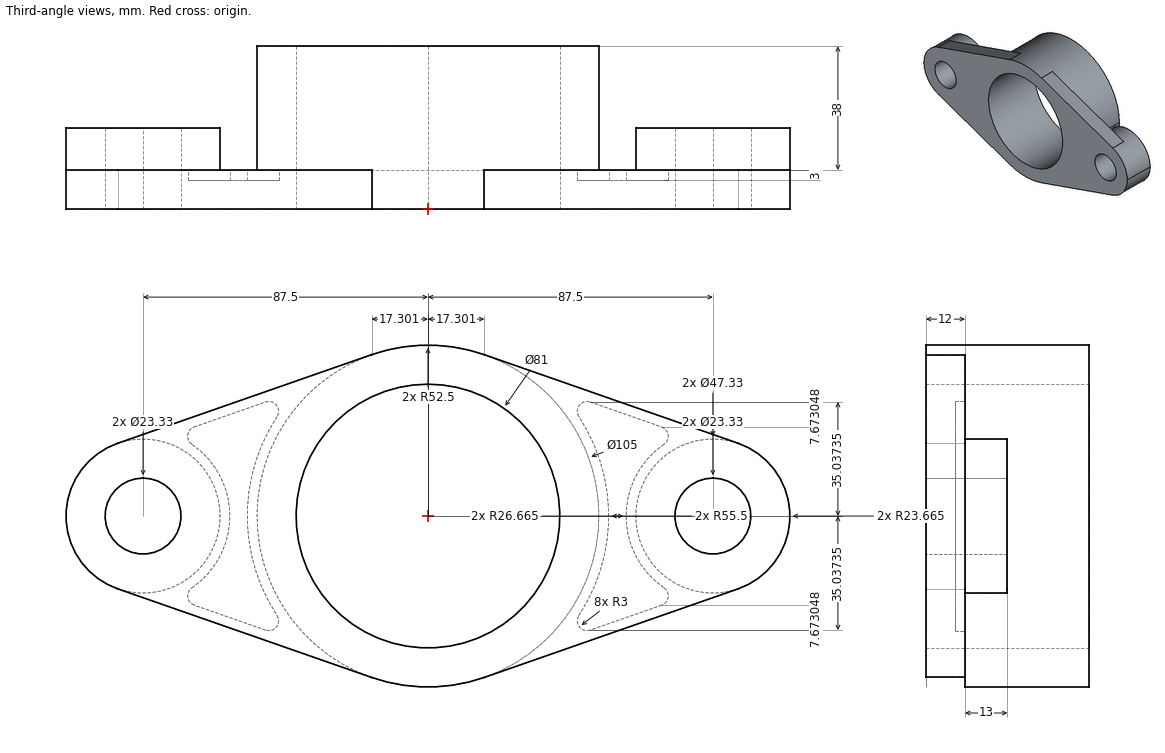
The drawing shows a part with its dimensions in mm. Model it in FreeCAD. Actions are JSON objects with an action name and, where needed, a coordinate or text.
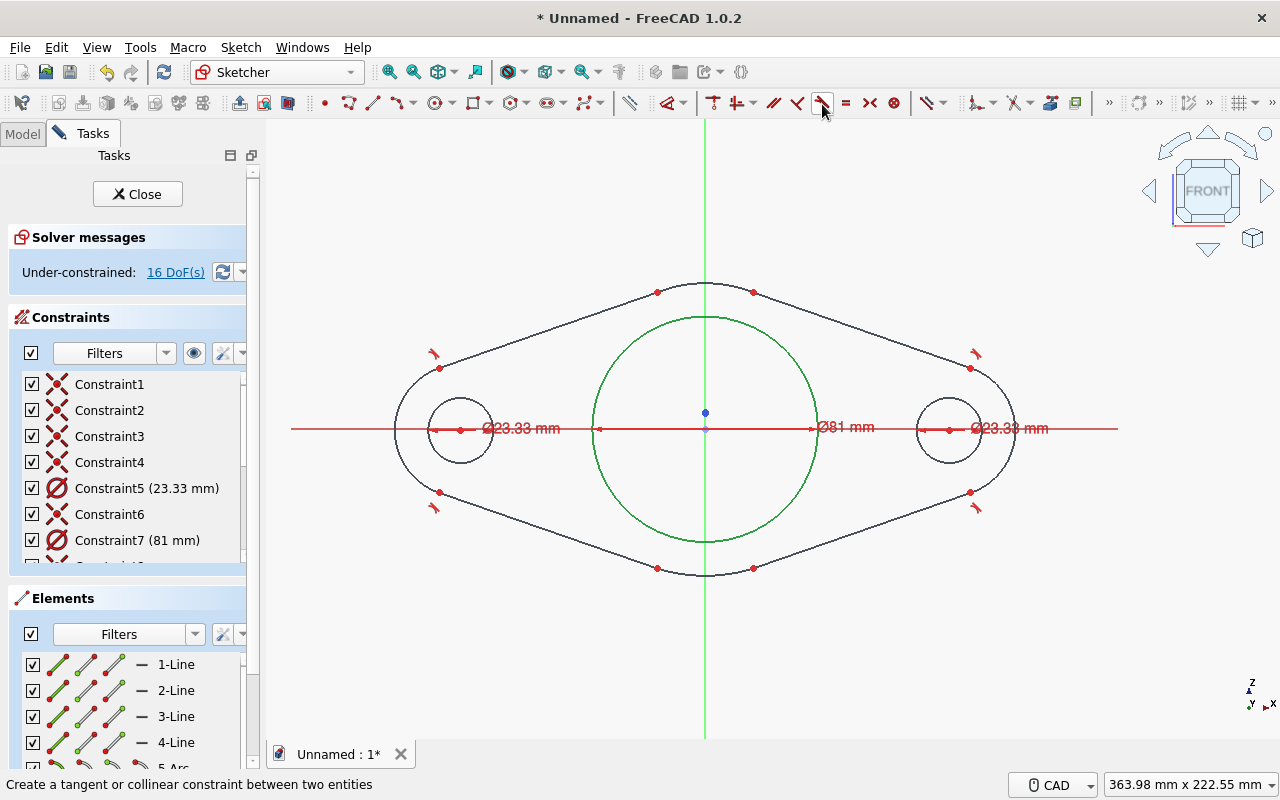
{"action": "left_click", "coordinate": [785, 349]}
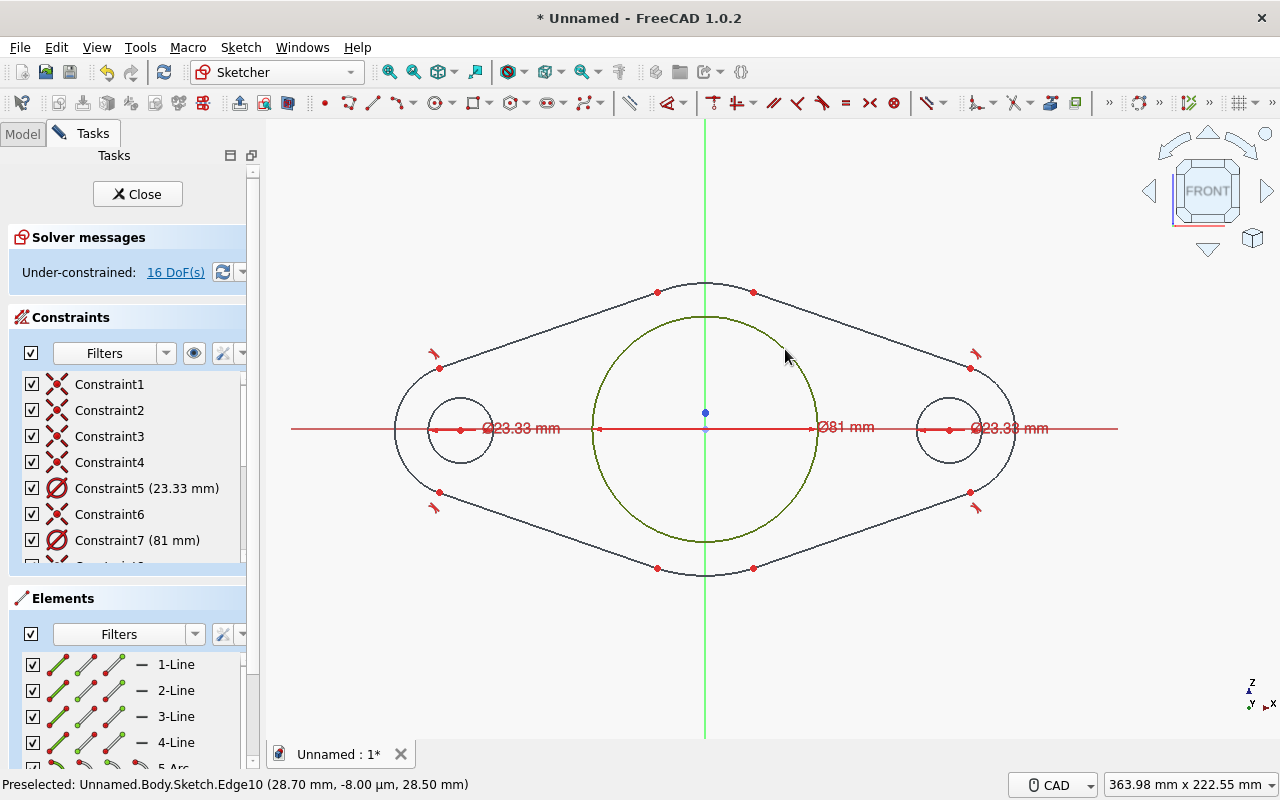
{"action": "left_click", "coordinate": [725, 285]}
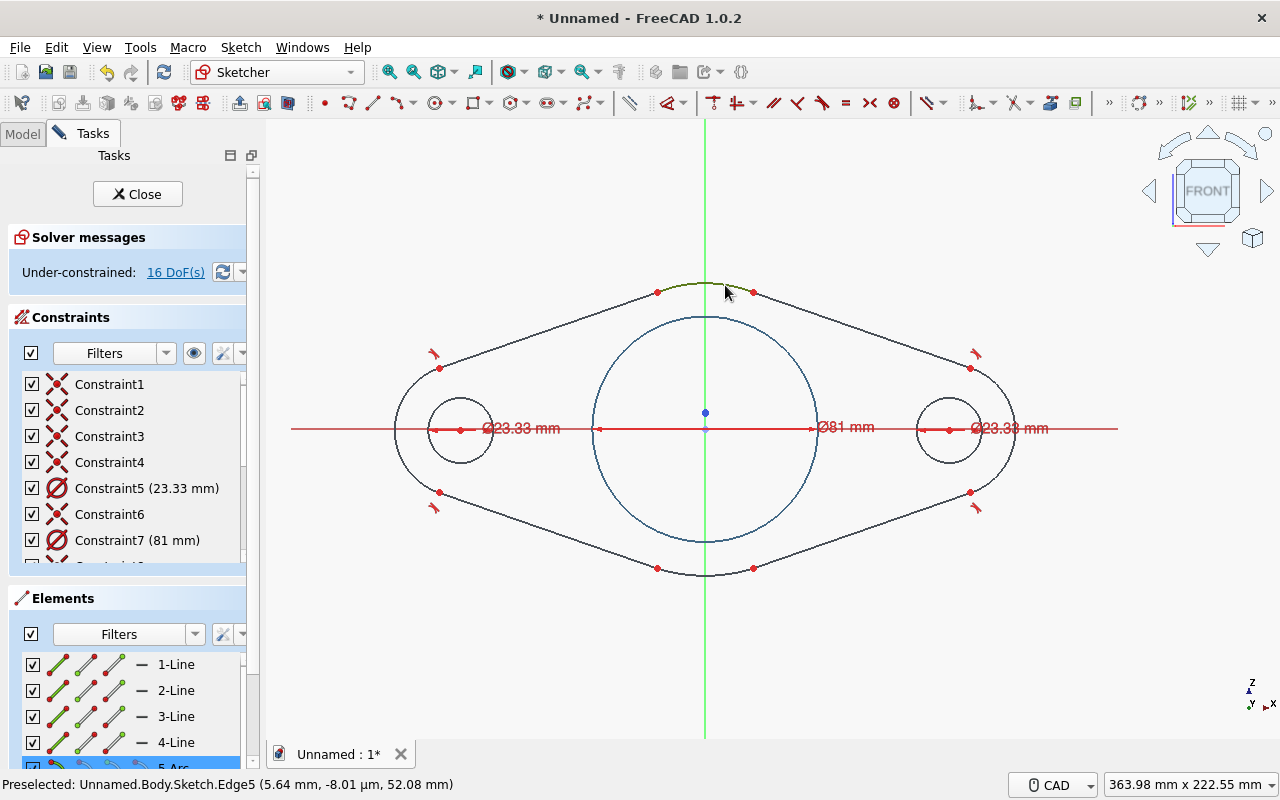
{"action": "left_click", "coordinate": [714, 104]}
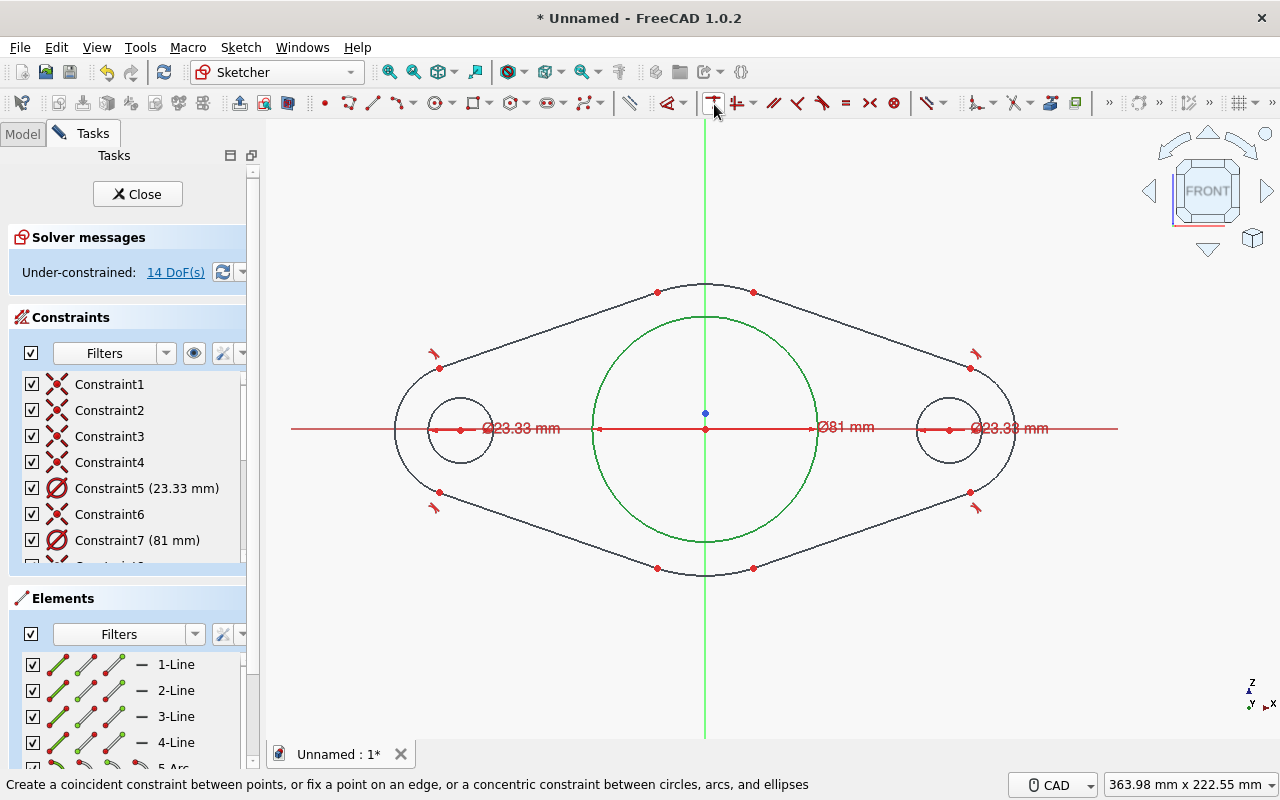
{"action": "left_click", "coordinate": [785, 349]}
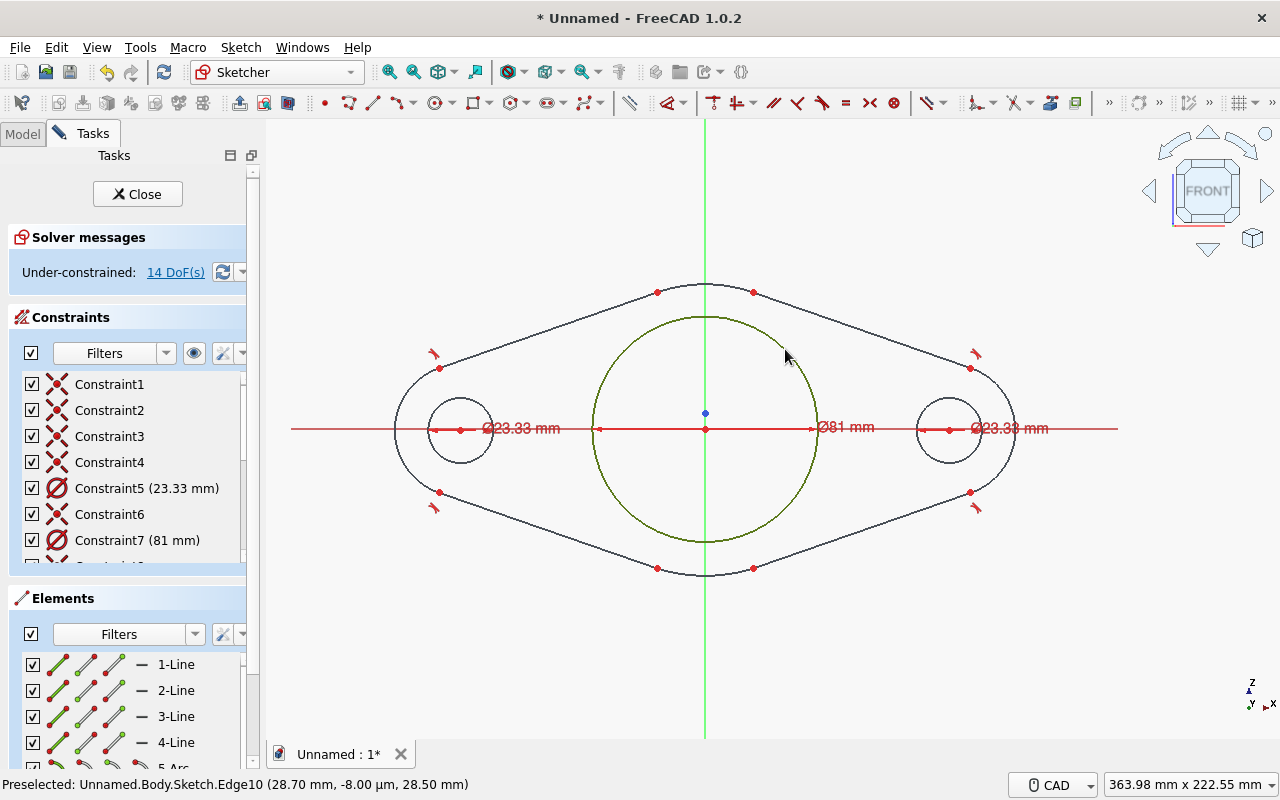
{"action": "left_click", "coordinate": [686, 575]}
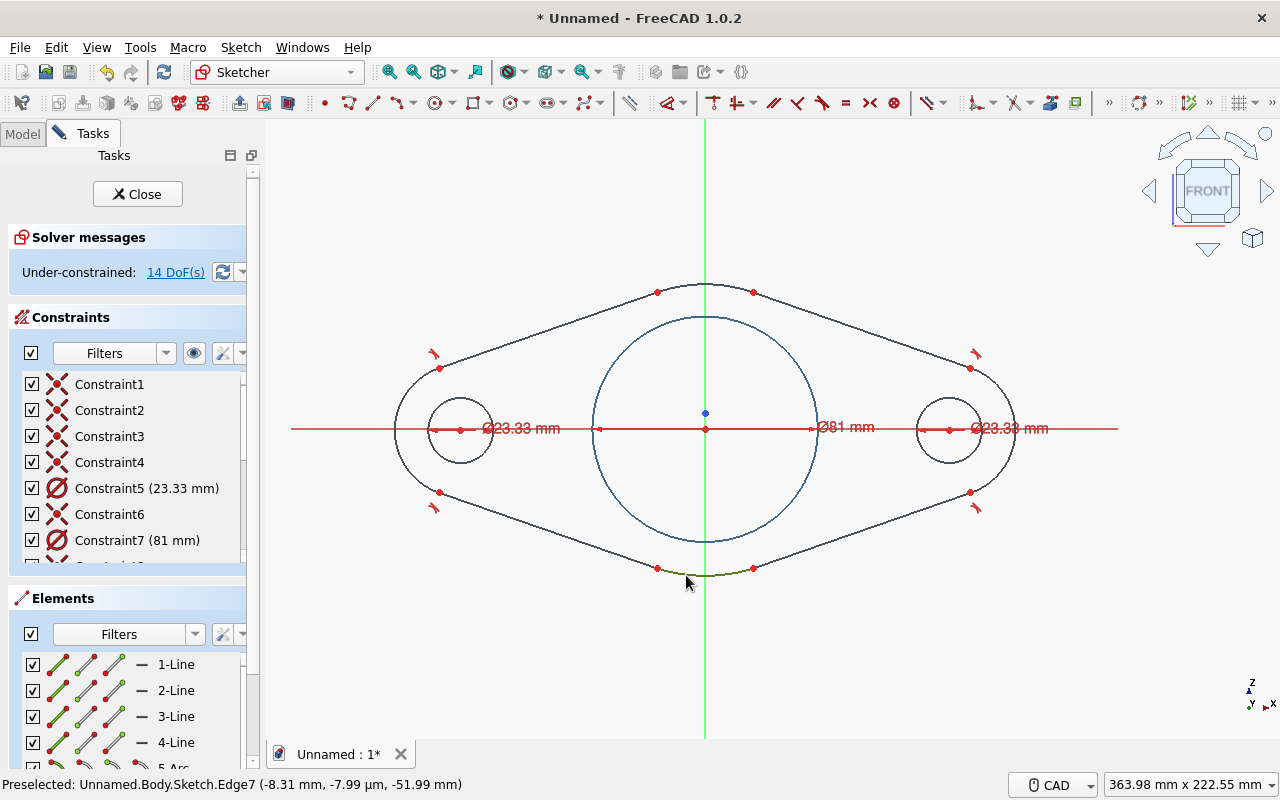
{"action": "left_click", "coordinate": [714, 104]}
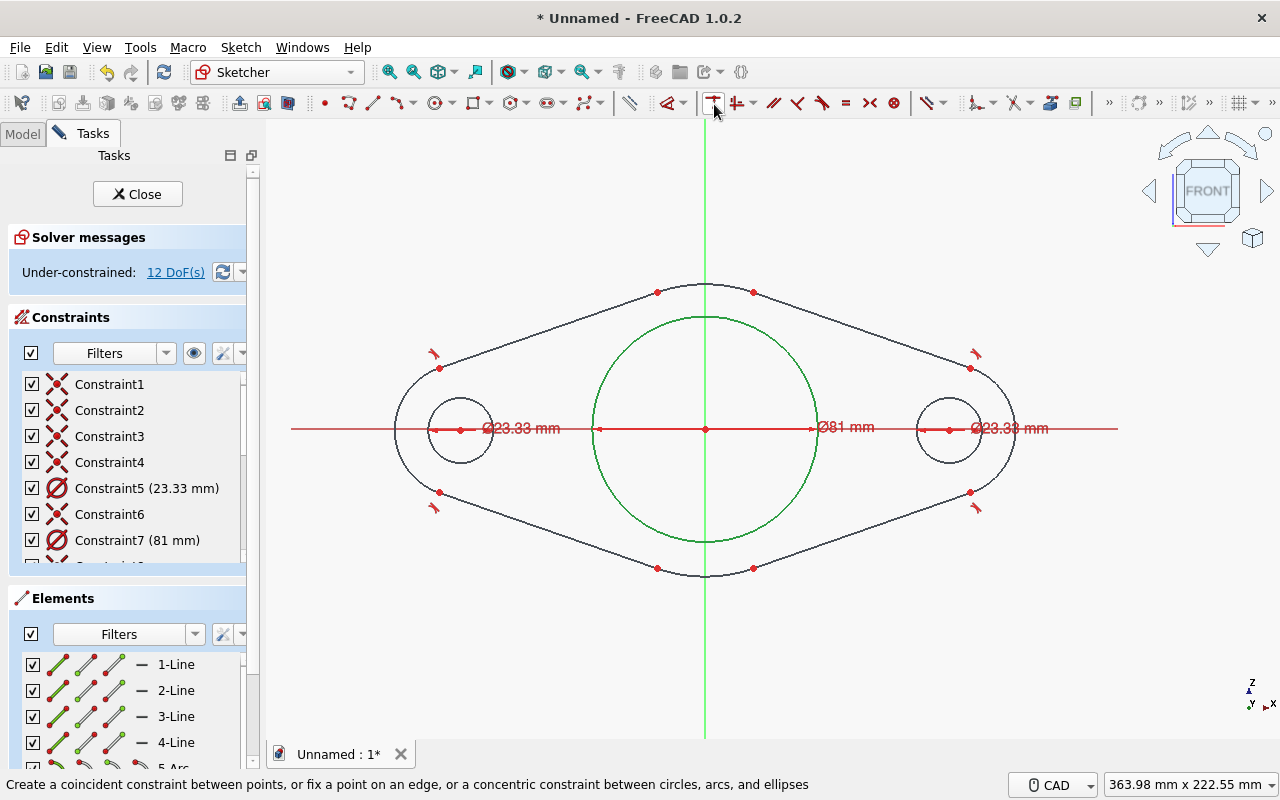
{"action": "left_click", "coordinate": [725, 286]}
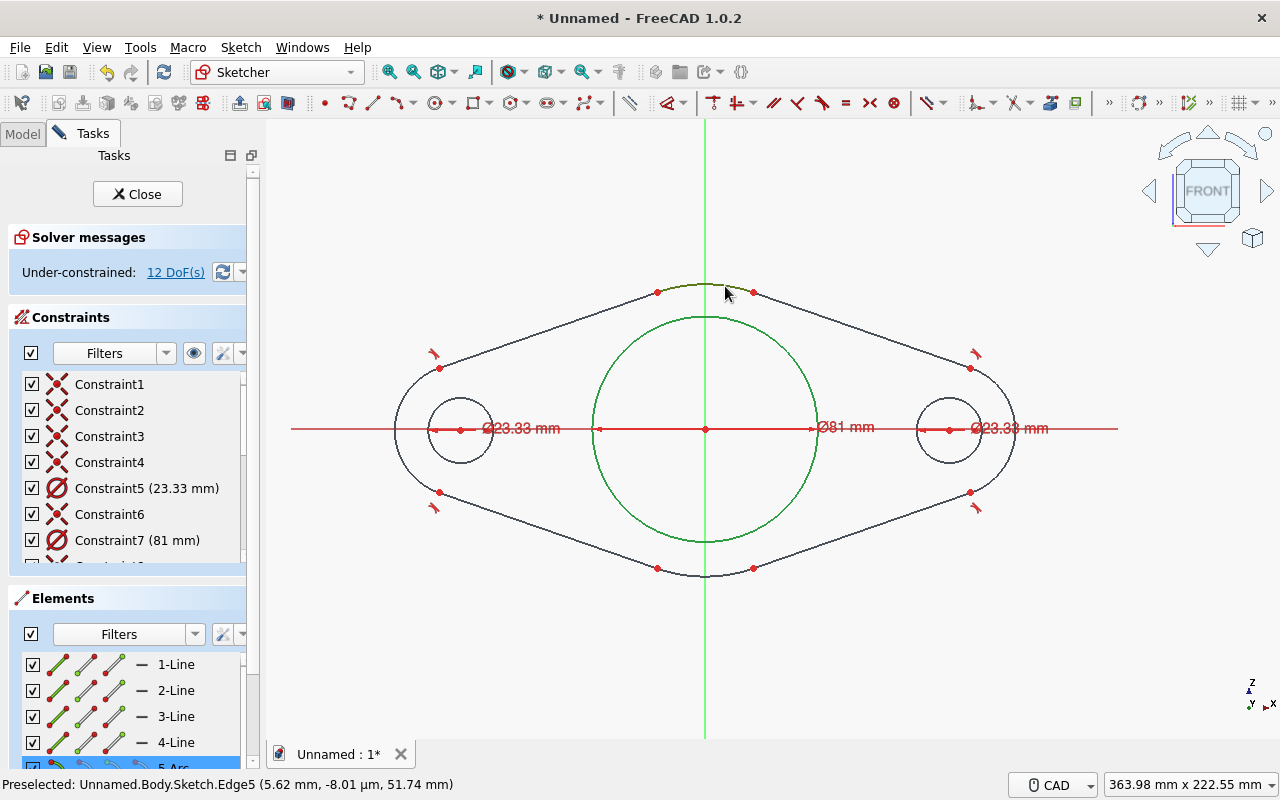
{"action": "left_click", "coordinate": [686, 575]}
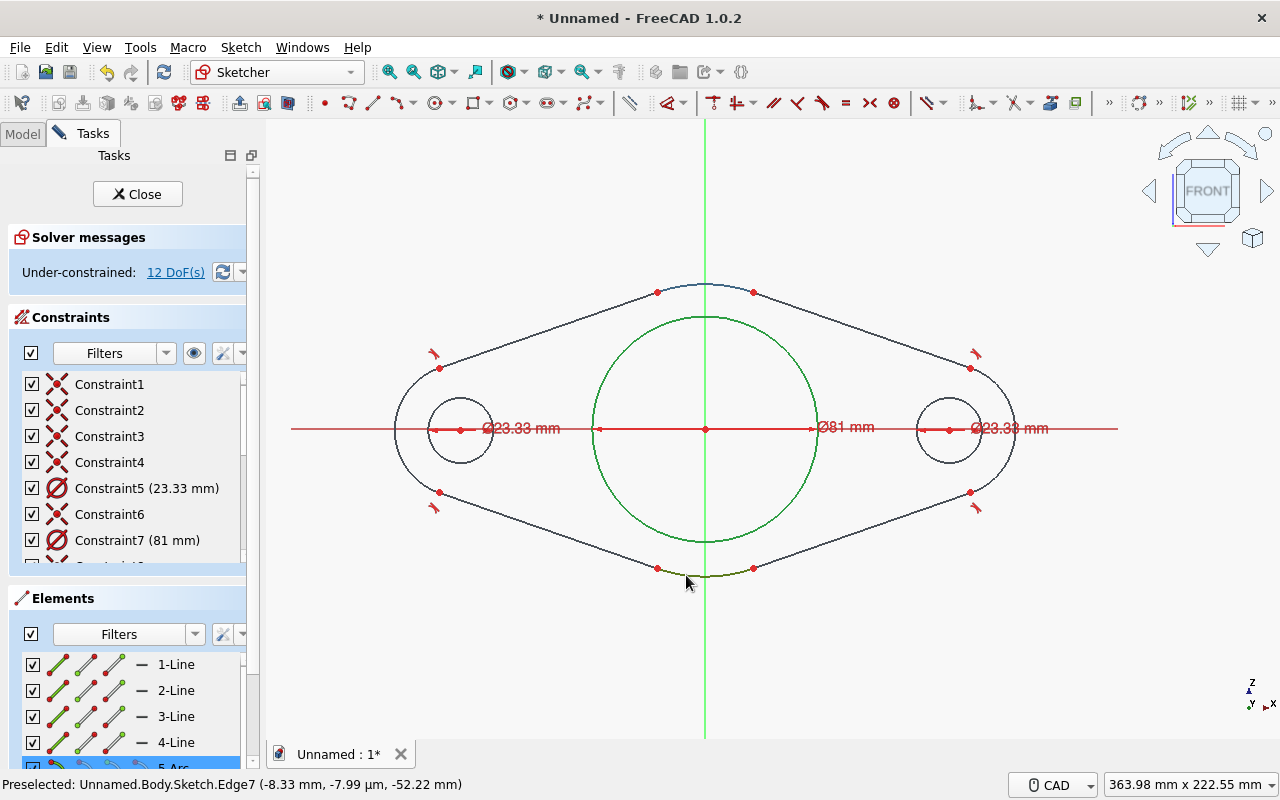
{"action": "left_click", "coordinate": [846, 104]}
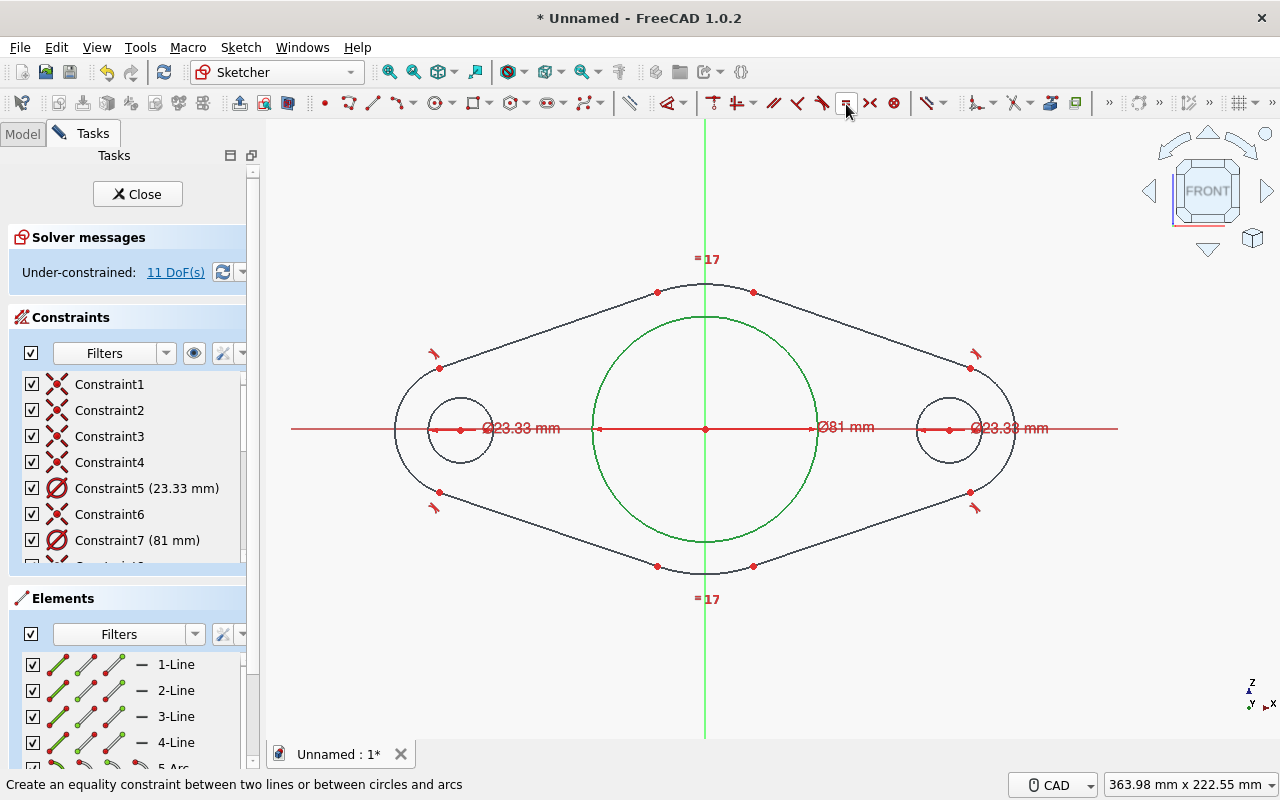
{"action": "left_click", "coordinate": [1007, 462]}